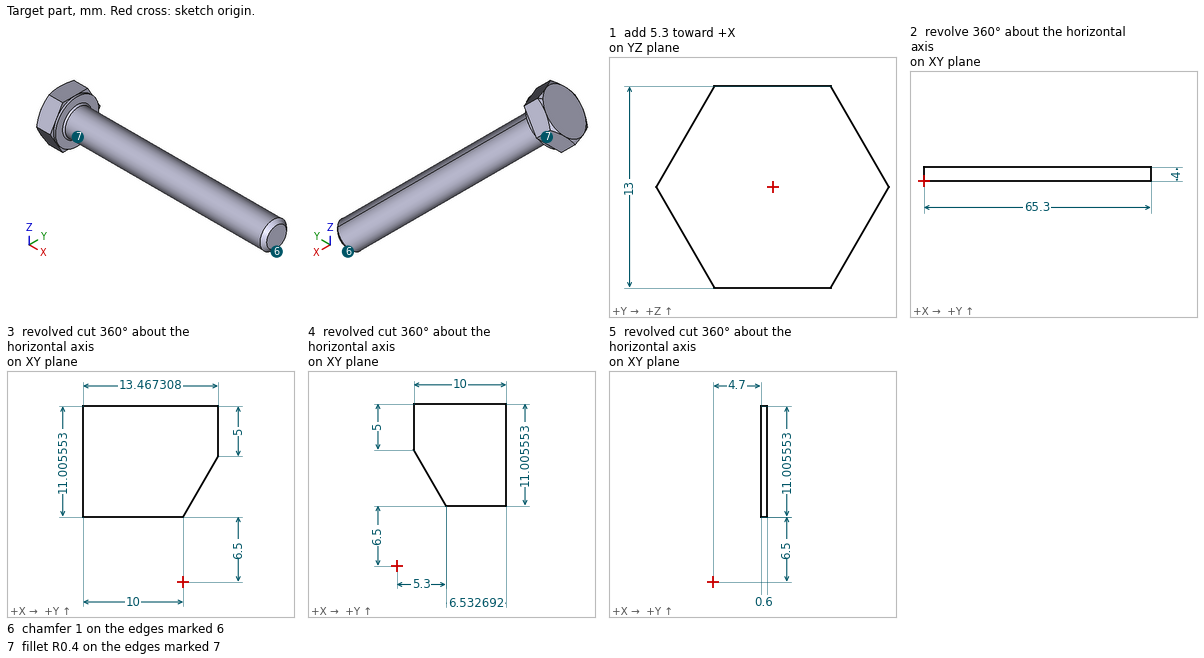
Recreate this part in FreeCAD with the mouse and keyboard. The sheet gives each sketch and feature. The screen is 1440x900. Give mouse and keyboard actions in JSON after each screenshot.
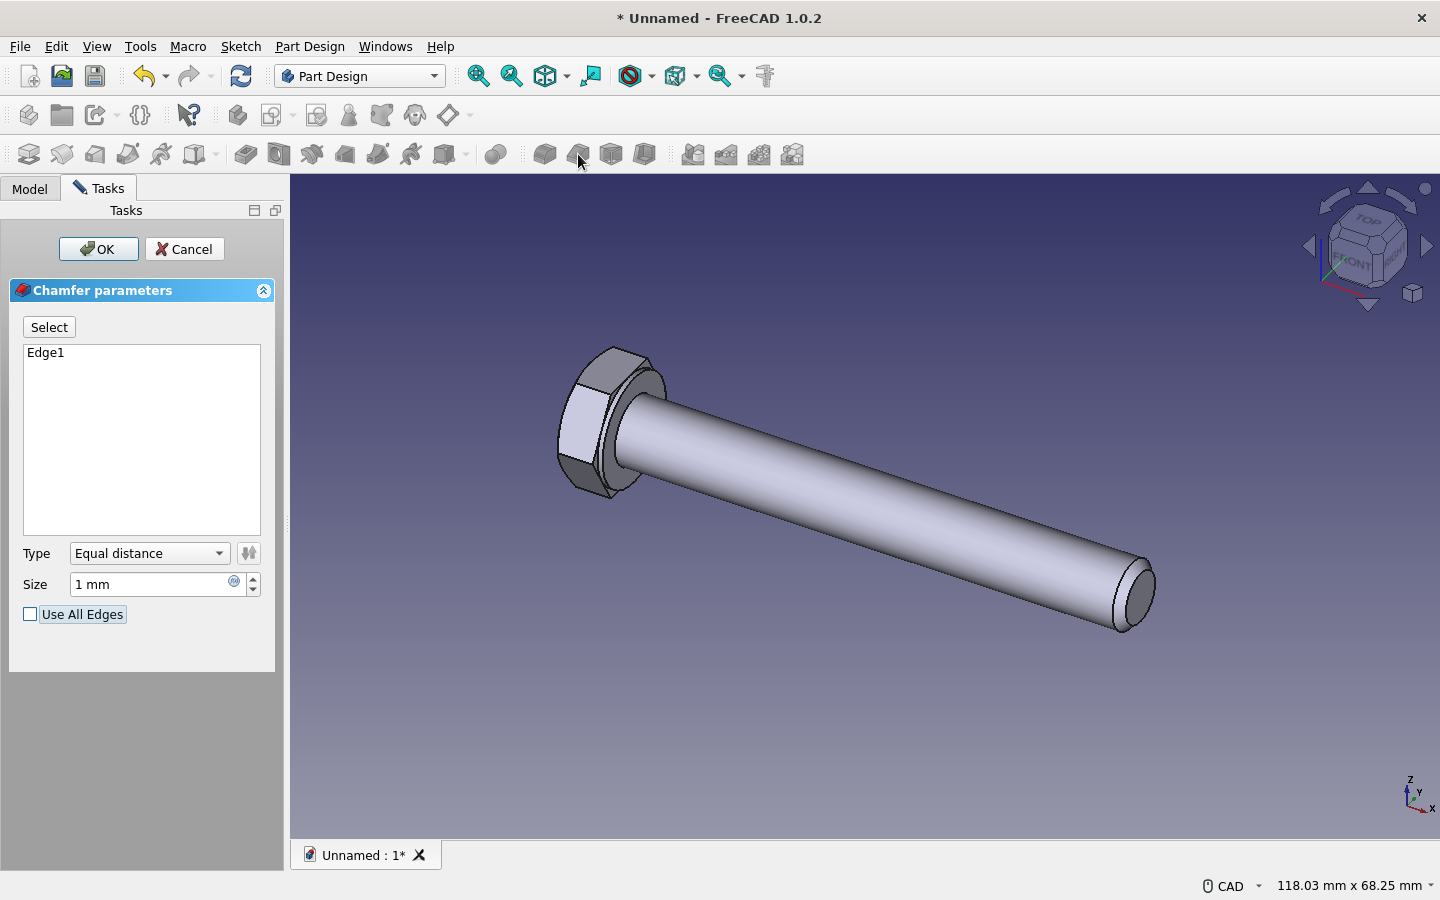
{"action": "left_click", "coordinate": [99, 249]}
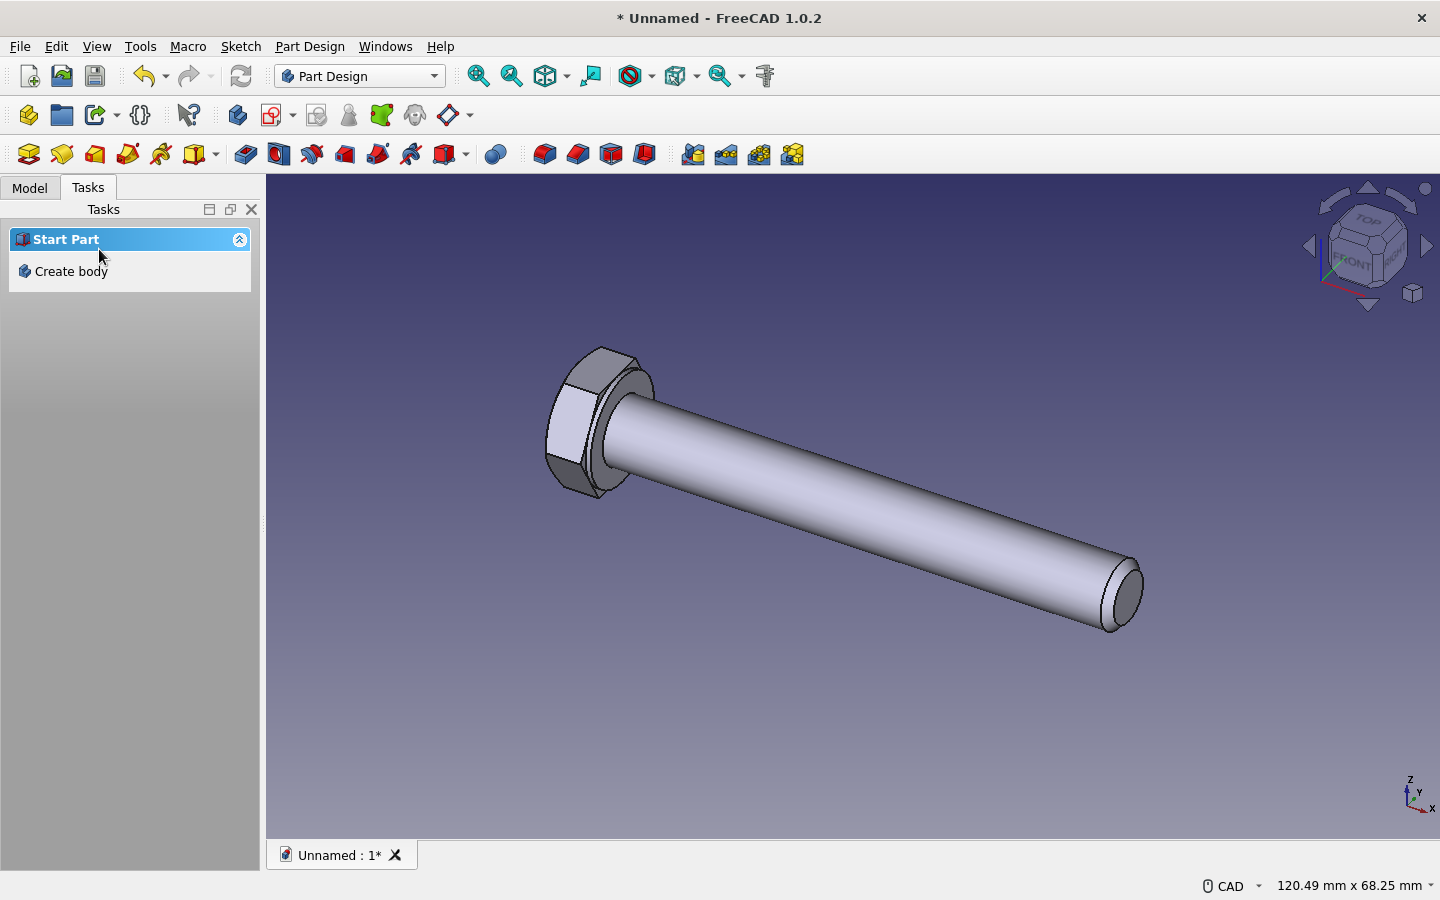
{"action": "key", "text": "0"}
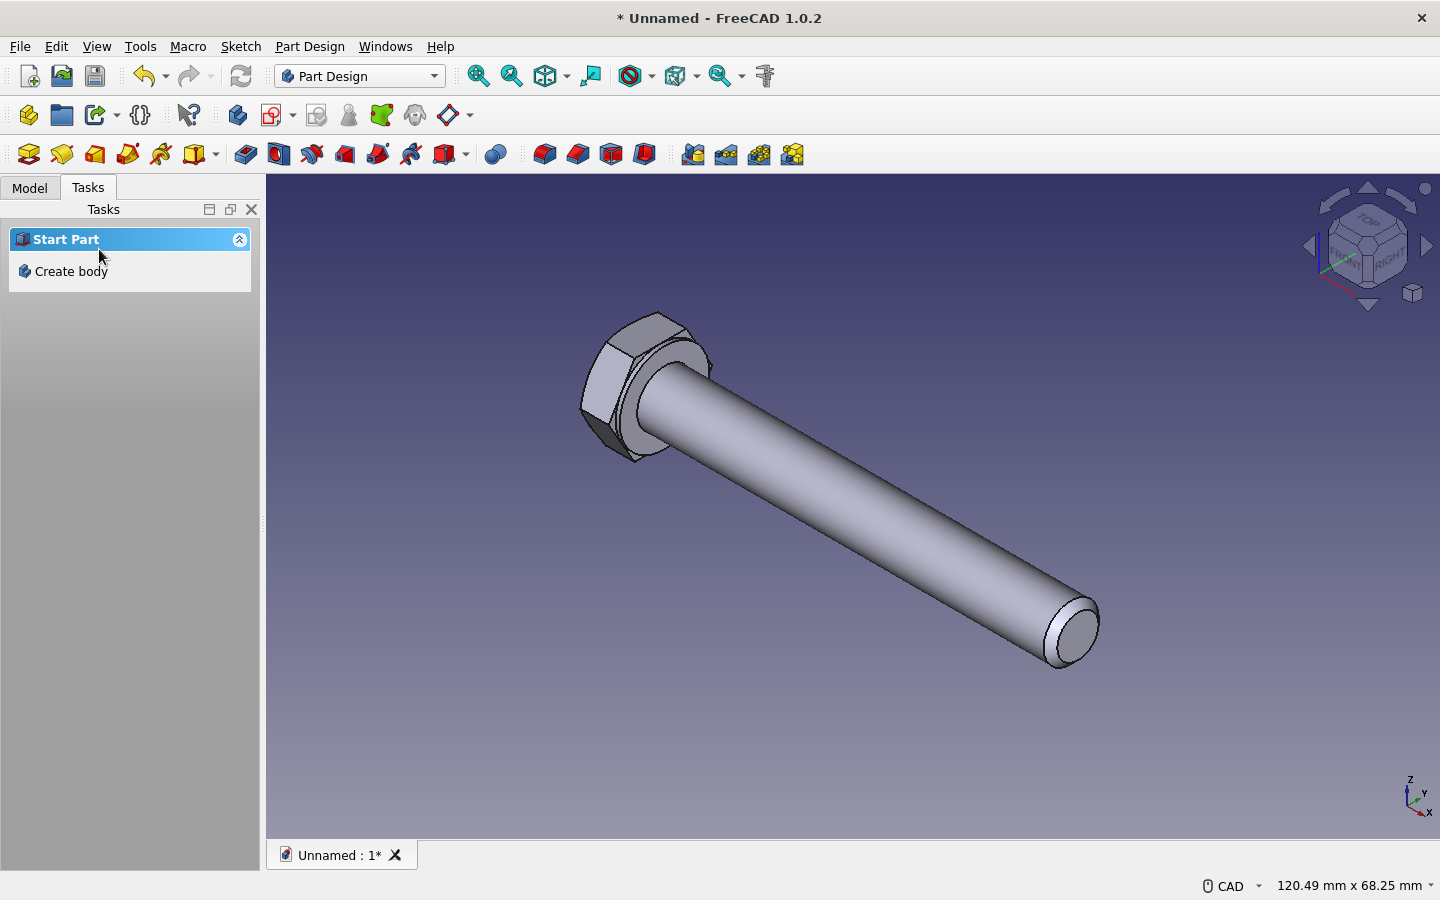
{"action": "key", "text": "2"}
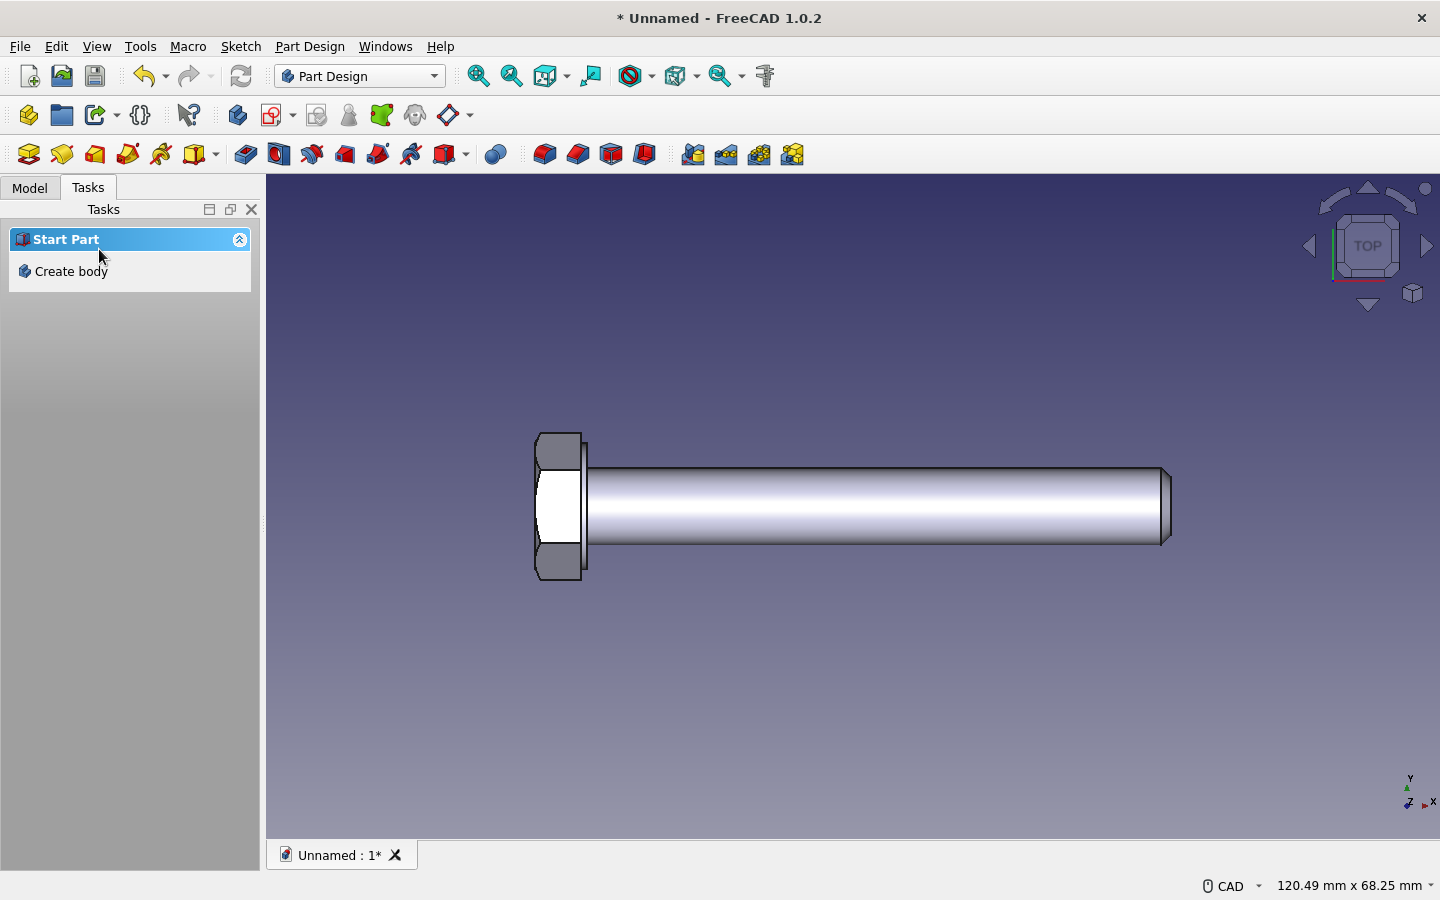
{"action": "key", "text": "1"}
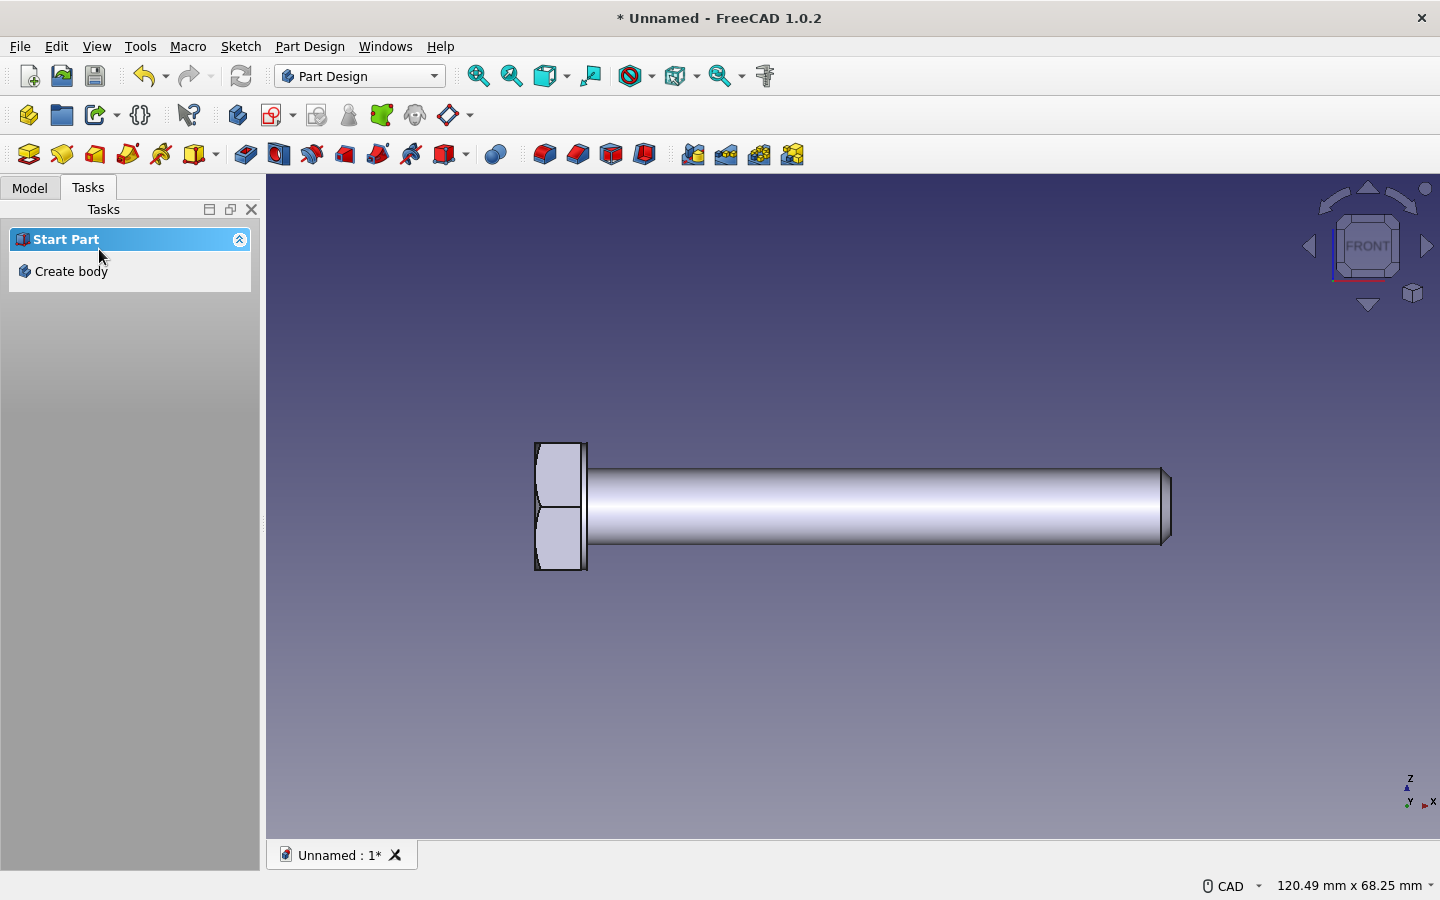
{"action": "key", "text": "3"}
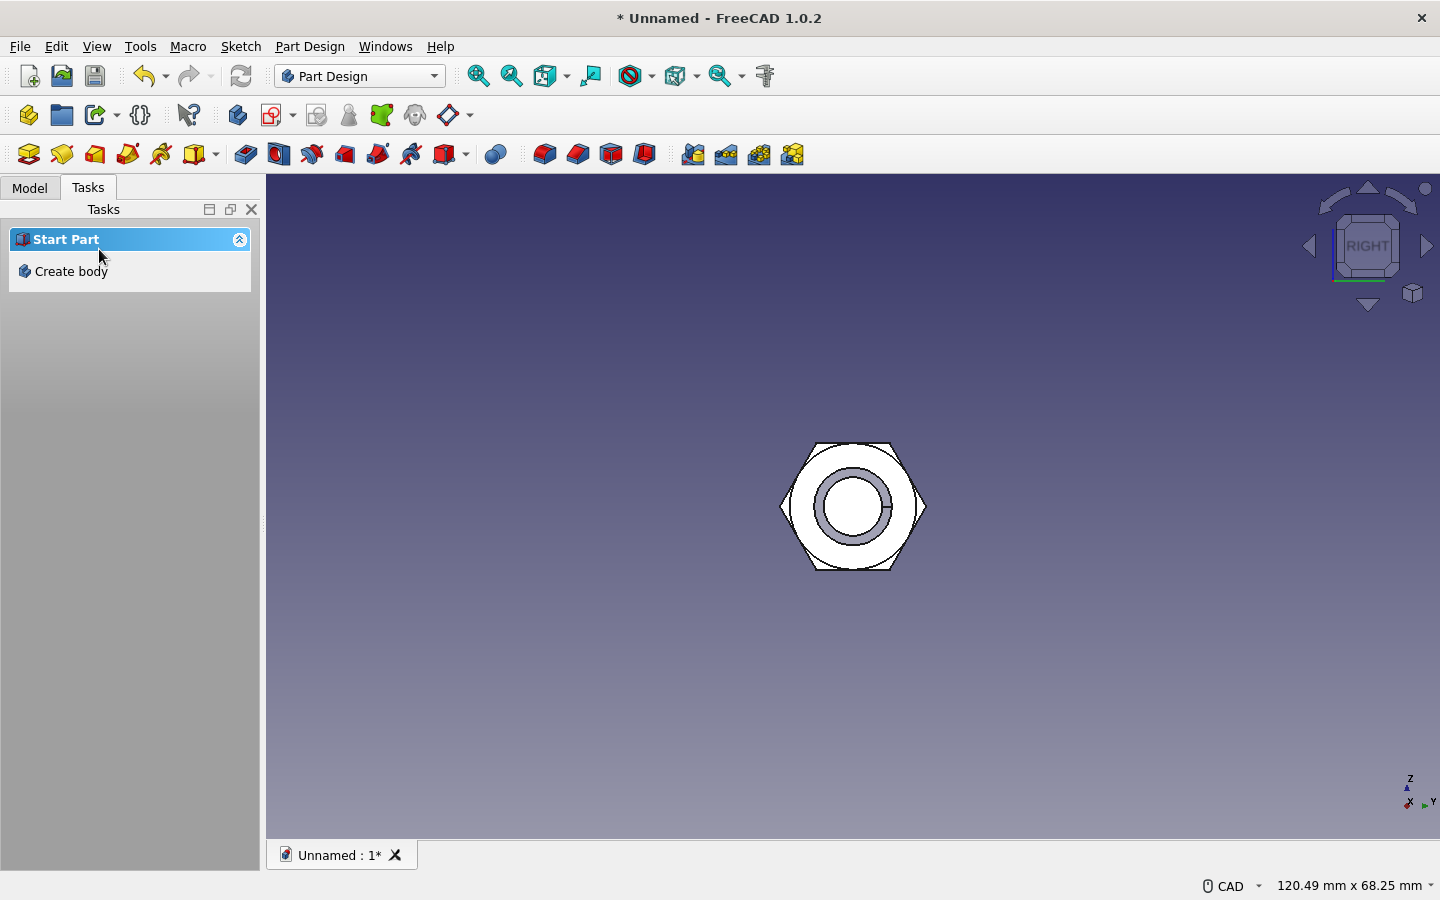
{"action": "left_click", "coordinate": [479, 76]}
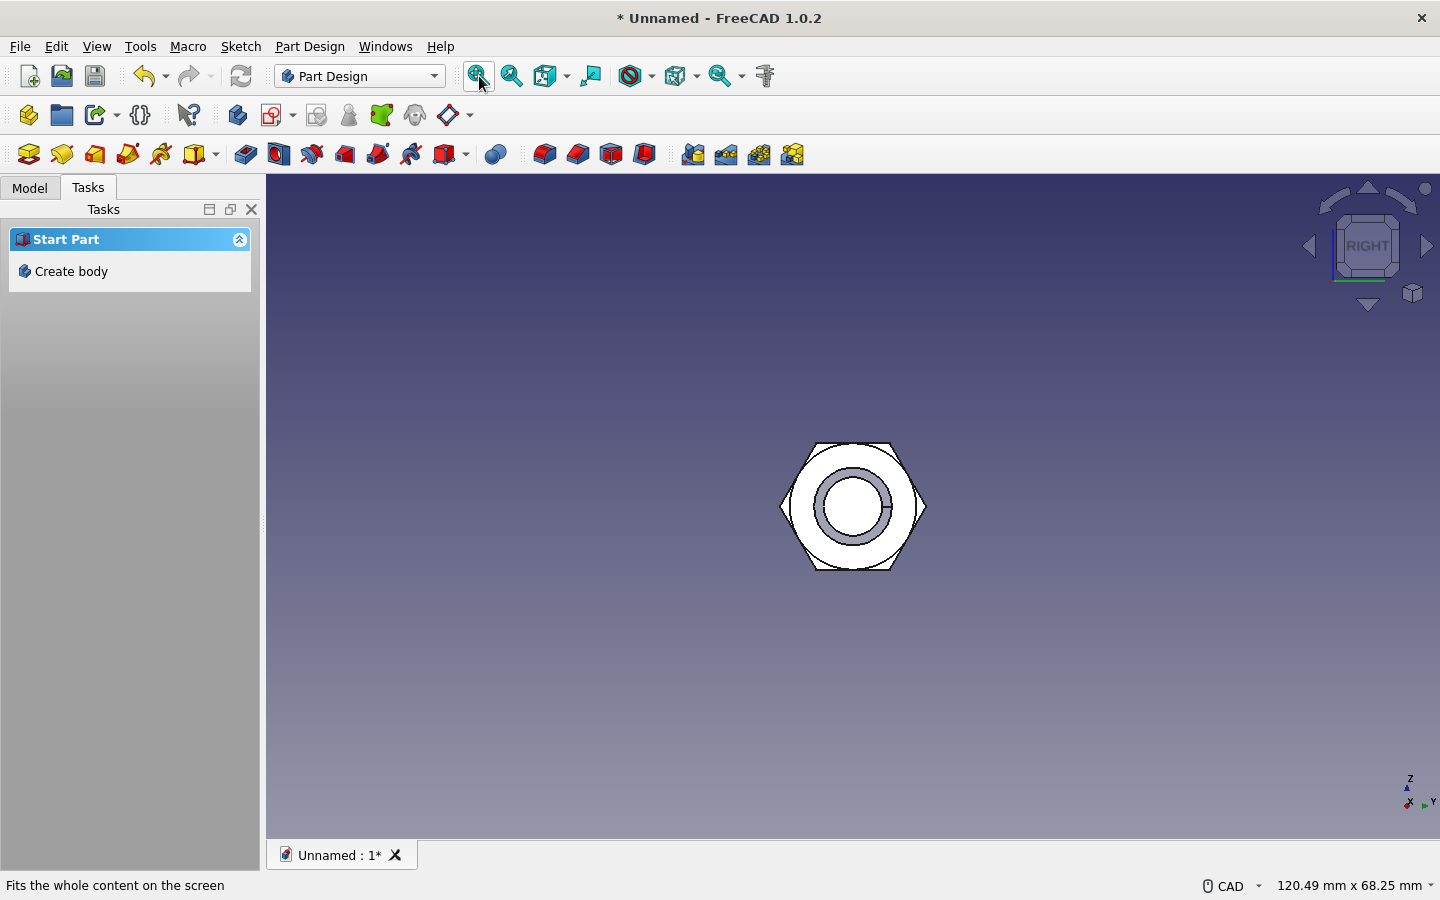
{"action": "key", "text": "5"}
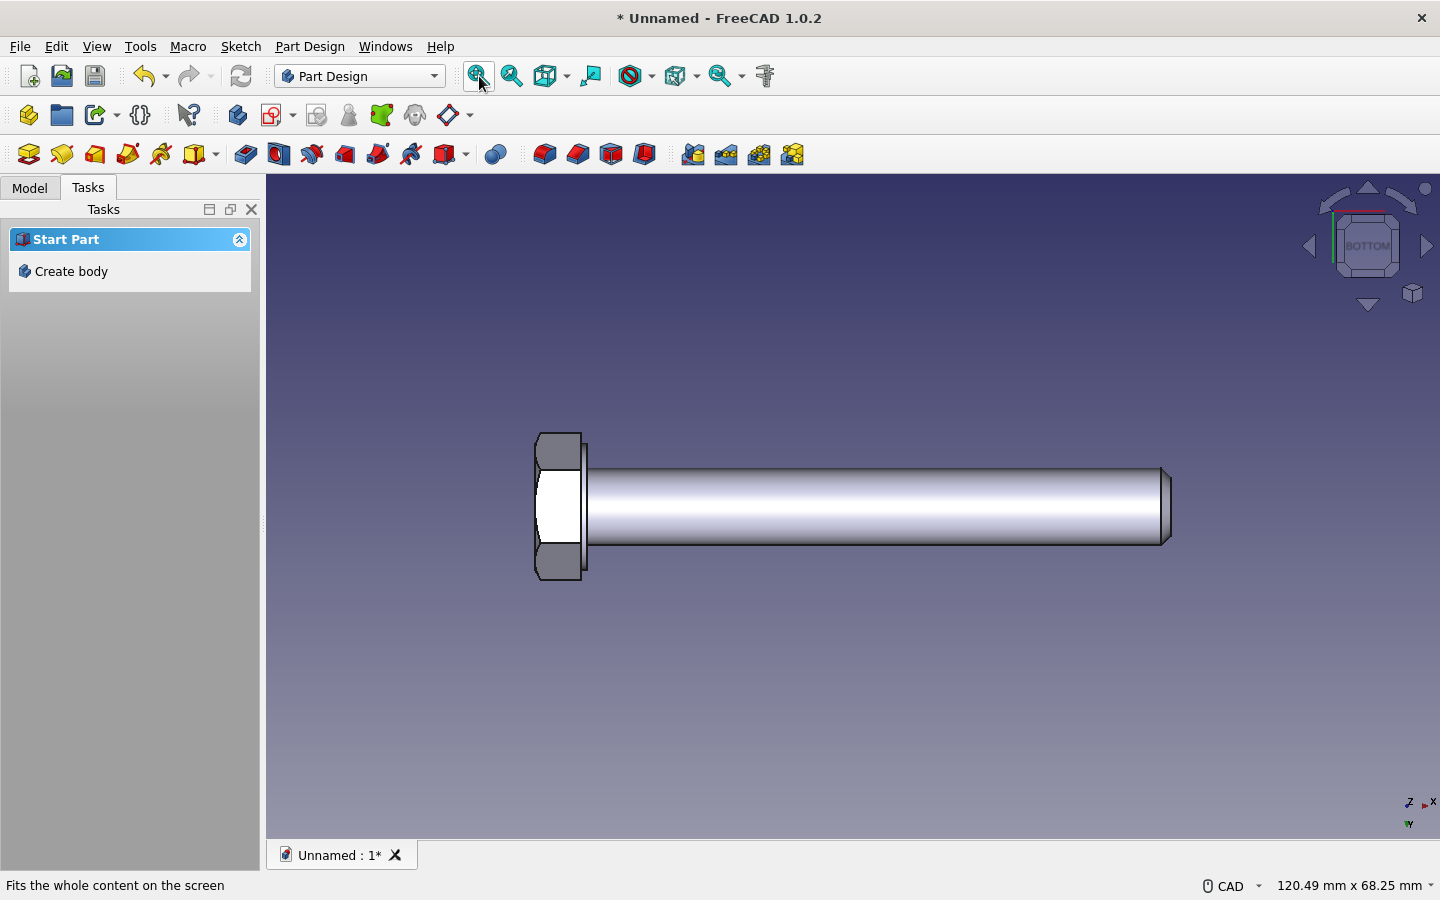
{"action": "key", "text": "4"}